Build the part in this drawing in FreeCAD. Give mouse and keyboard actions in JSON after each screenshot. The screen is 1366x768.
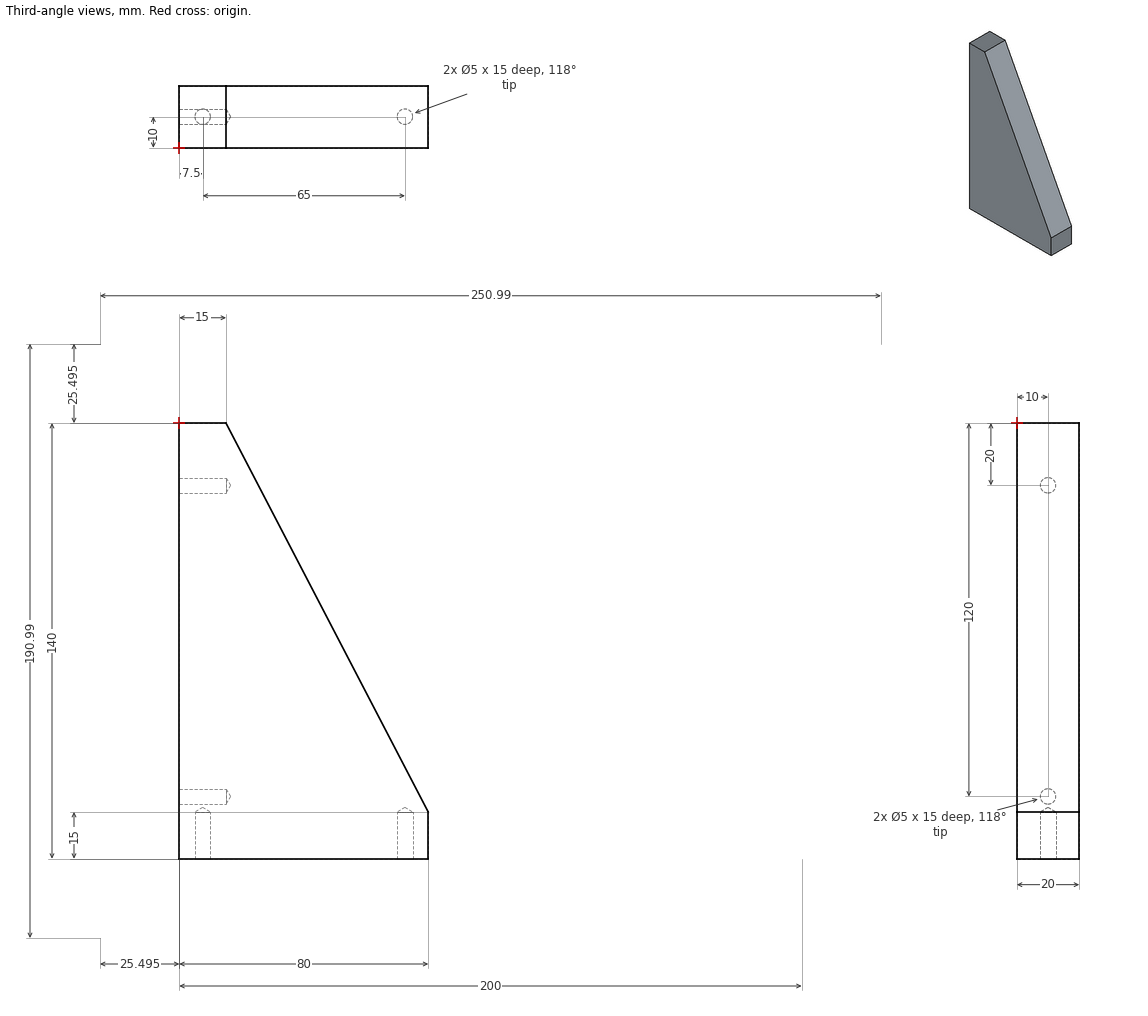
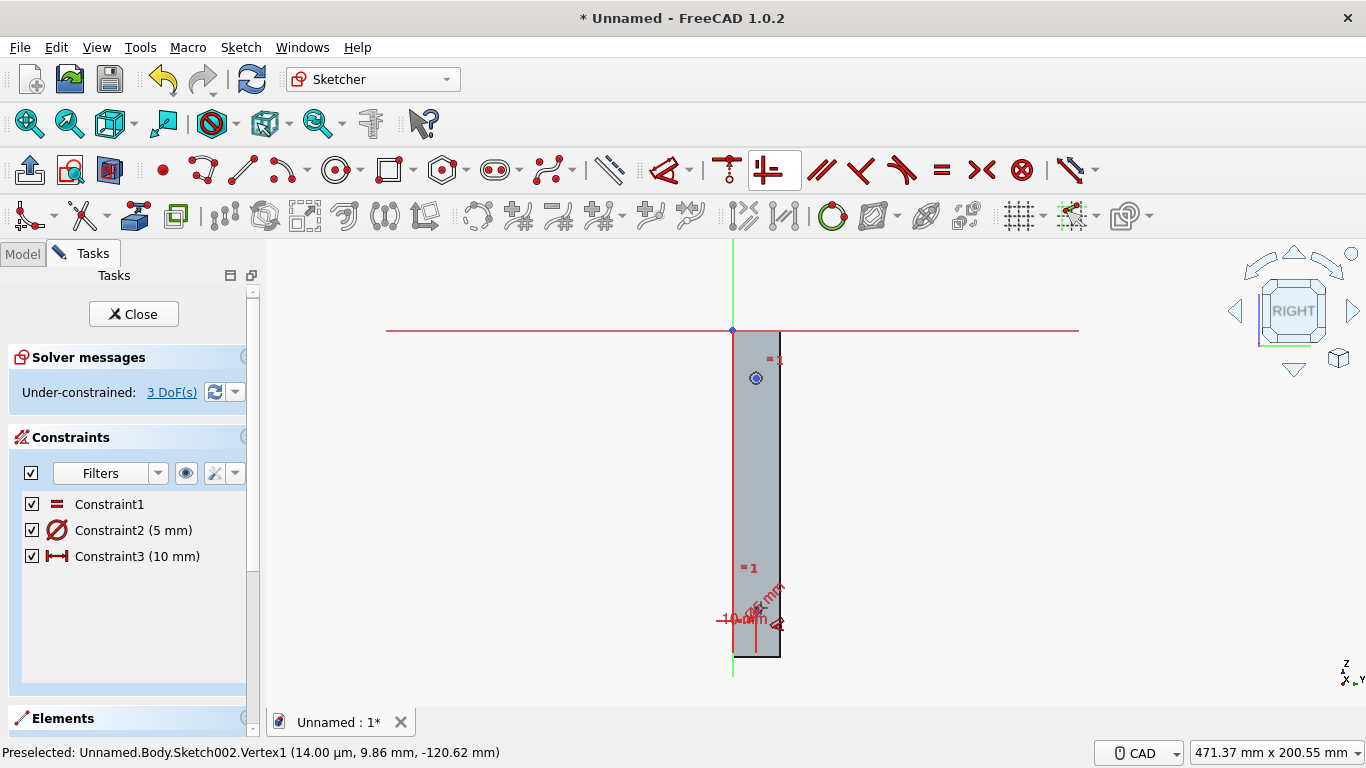
{"action": "scroll", "coordinate": [756, 378], "scroll_direction": "up", "scroll_amount": 3}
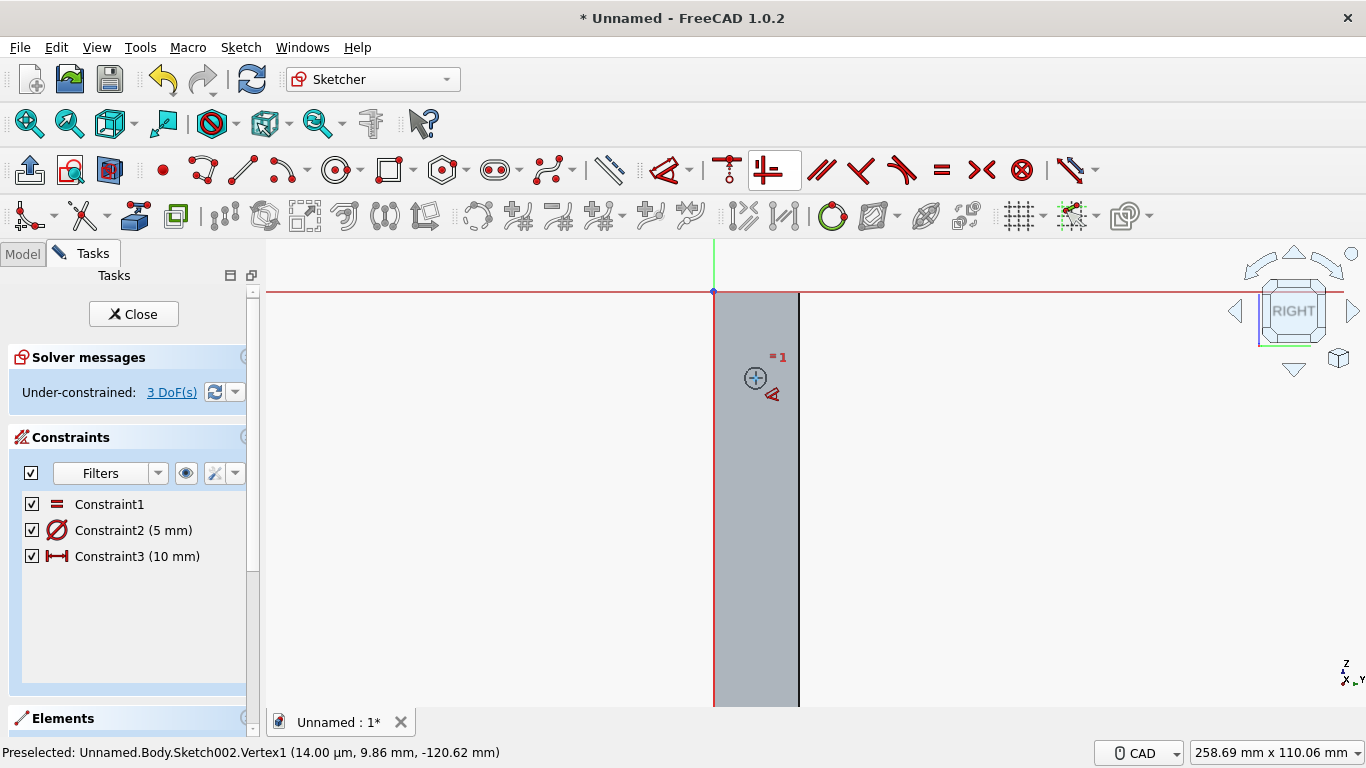
{"action": "left_click", "coordinate": [756, 378]}
{"action": "left_click", "coordinate": [735, 412]}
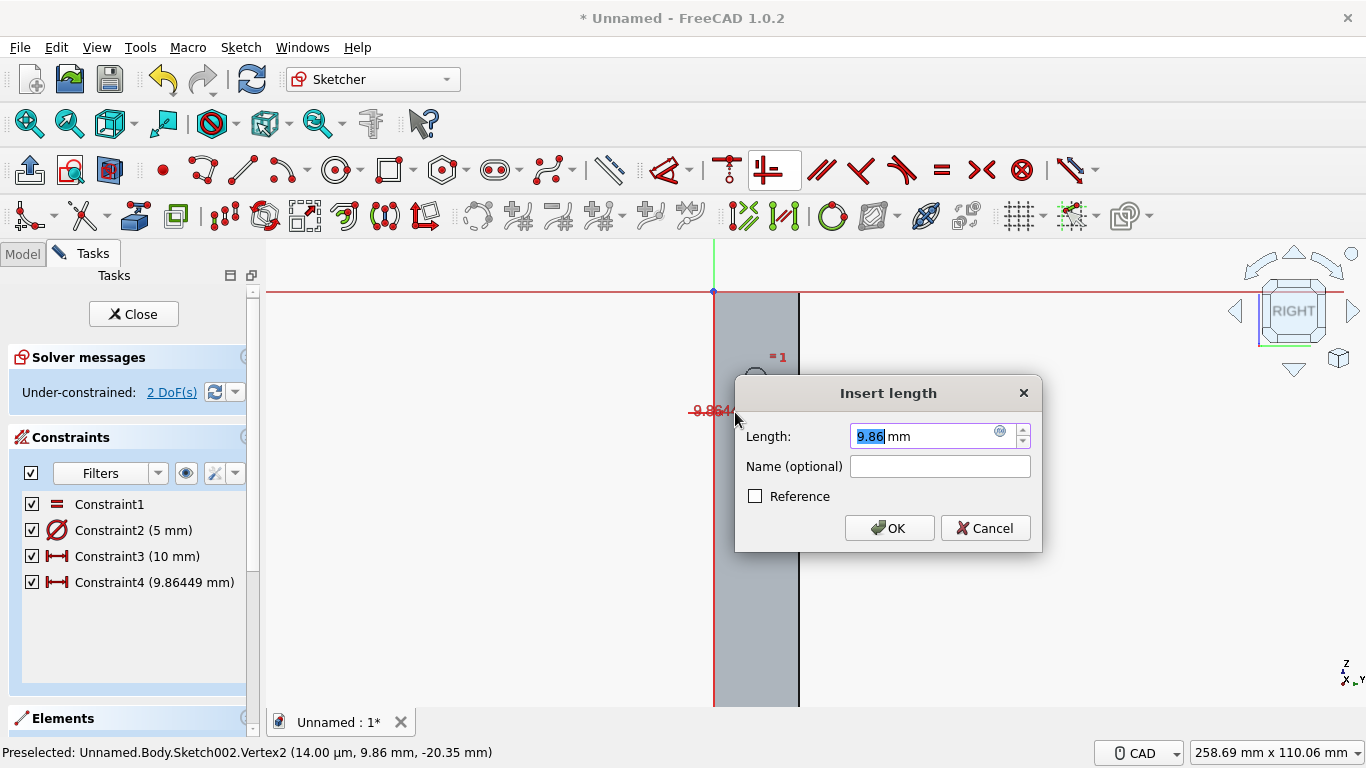
{"action": "type", "text": "10"}
{"action": "key", "text": "Return"}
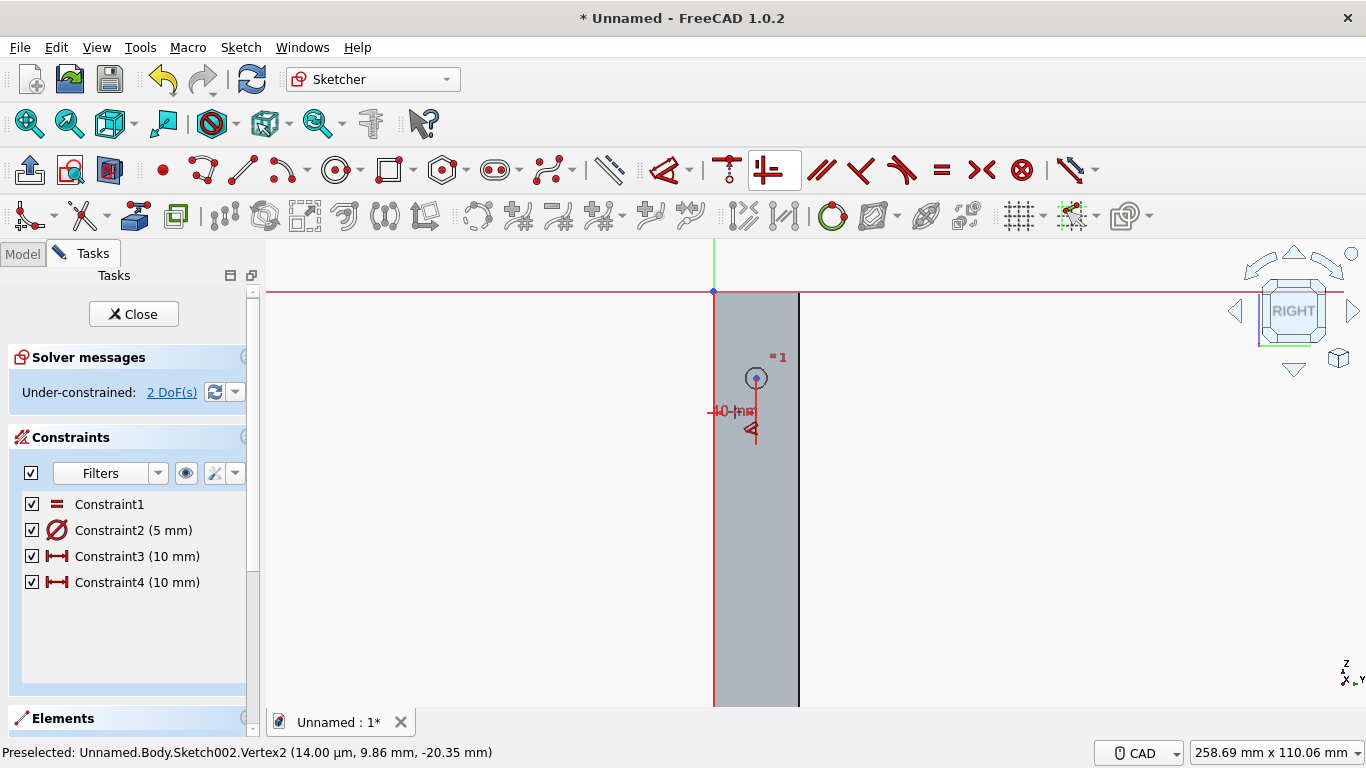
{"action": "left_click", "coordinate": [756, 378]}
{"action": "left_click", "coordinate": [680, 335]}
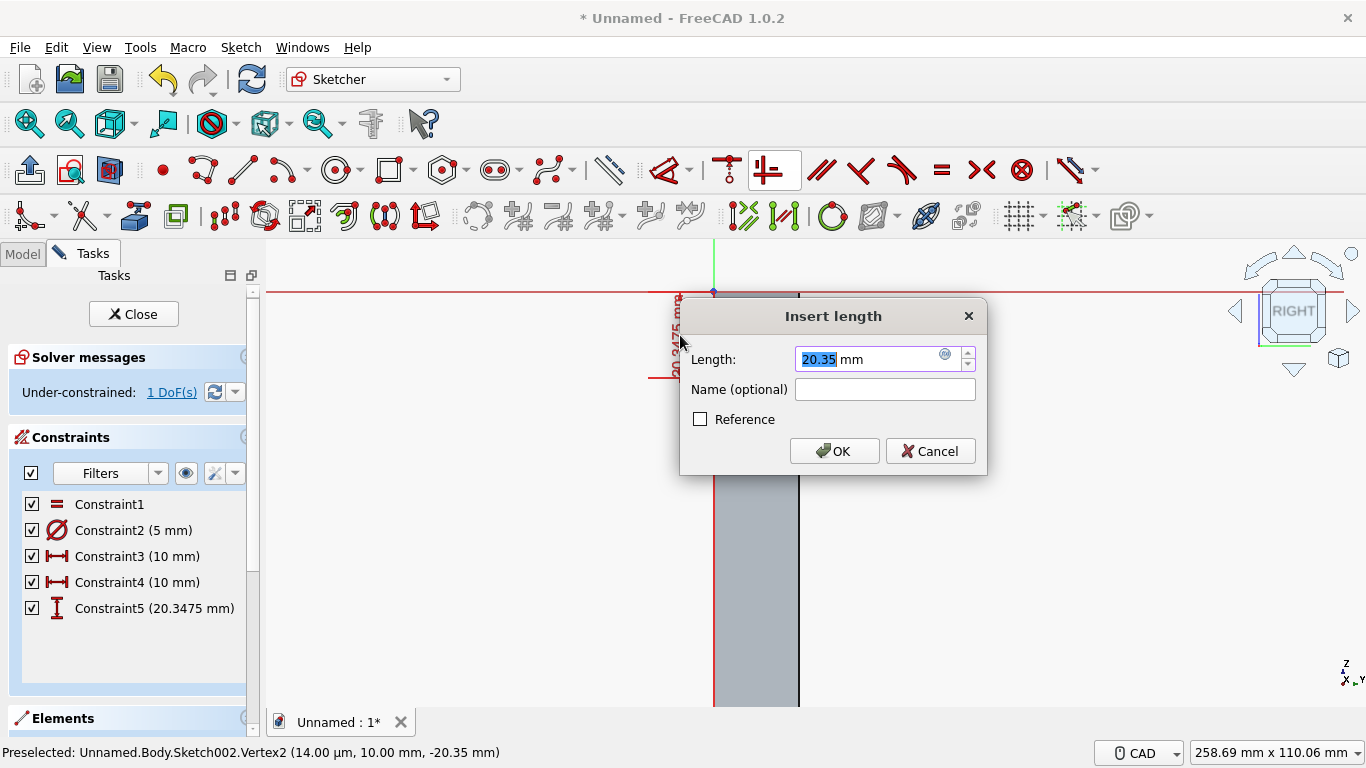
{"action": "type", "text": "20"}
{"action": "key", "text": "Return"}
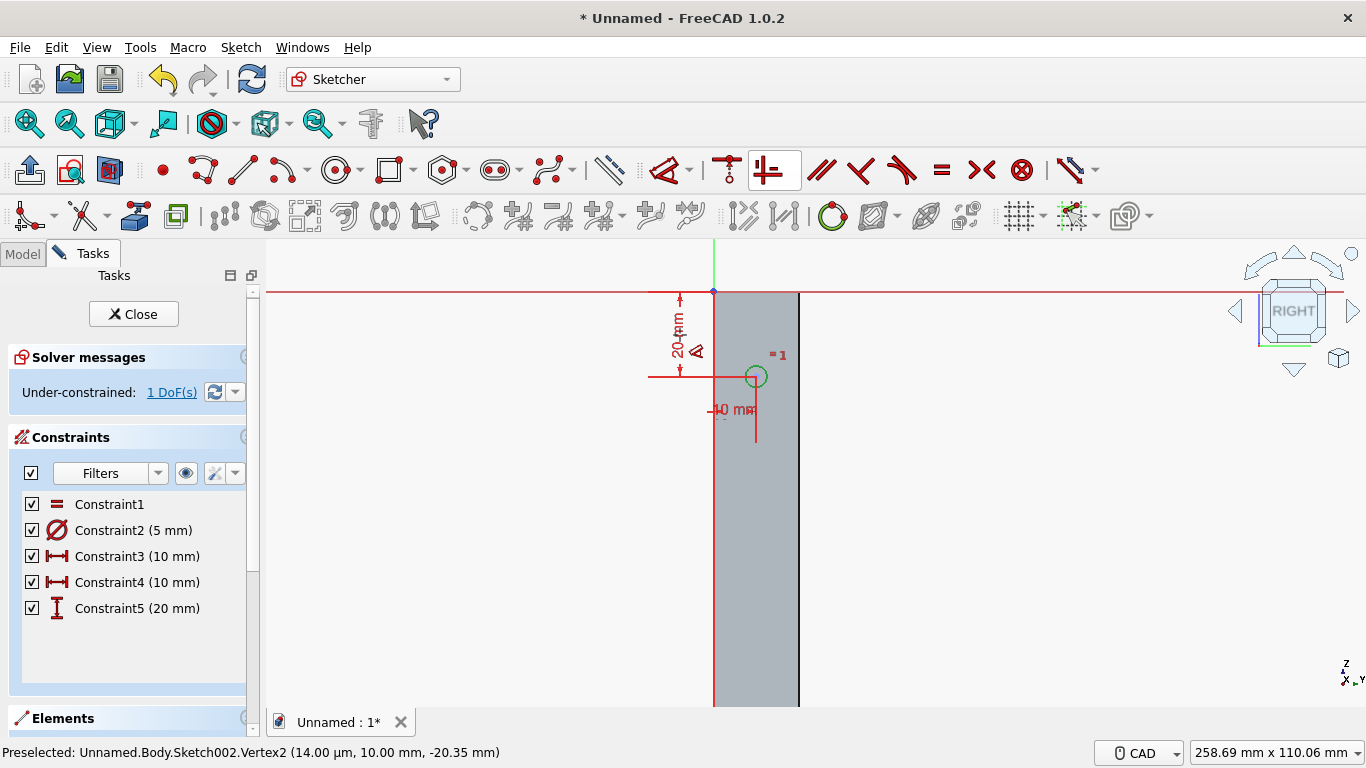
{"action": "scroll", "coordinate": [756, 377], "scroll_direction": "down", "scroll_amount": 3}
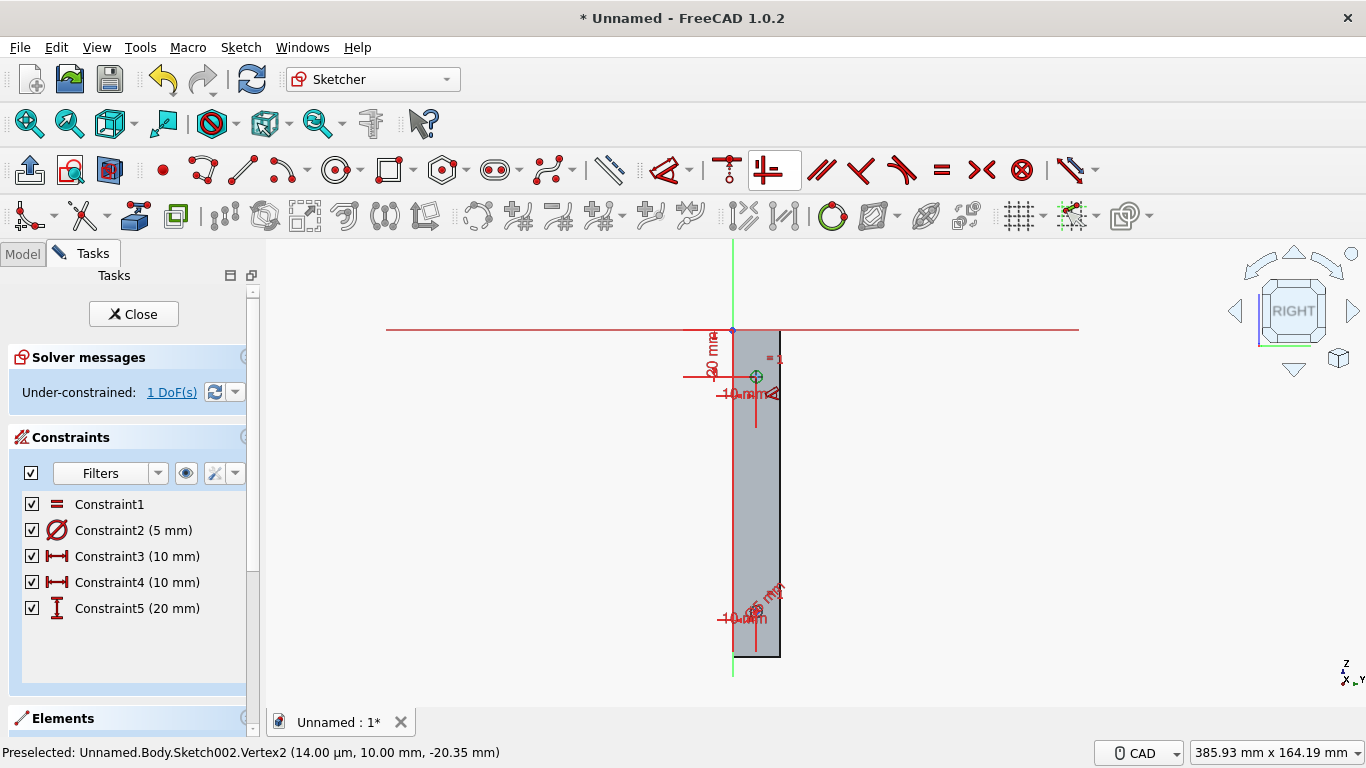
{"action": "left_click", "coordinate": [756, 612]}
{"action": "left_click", "coordinate": [699, 471]}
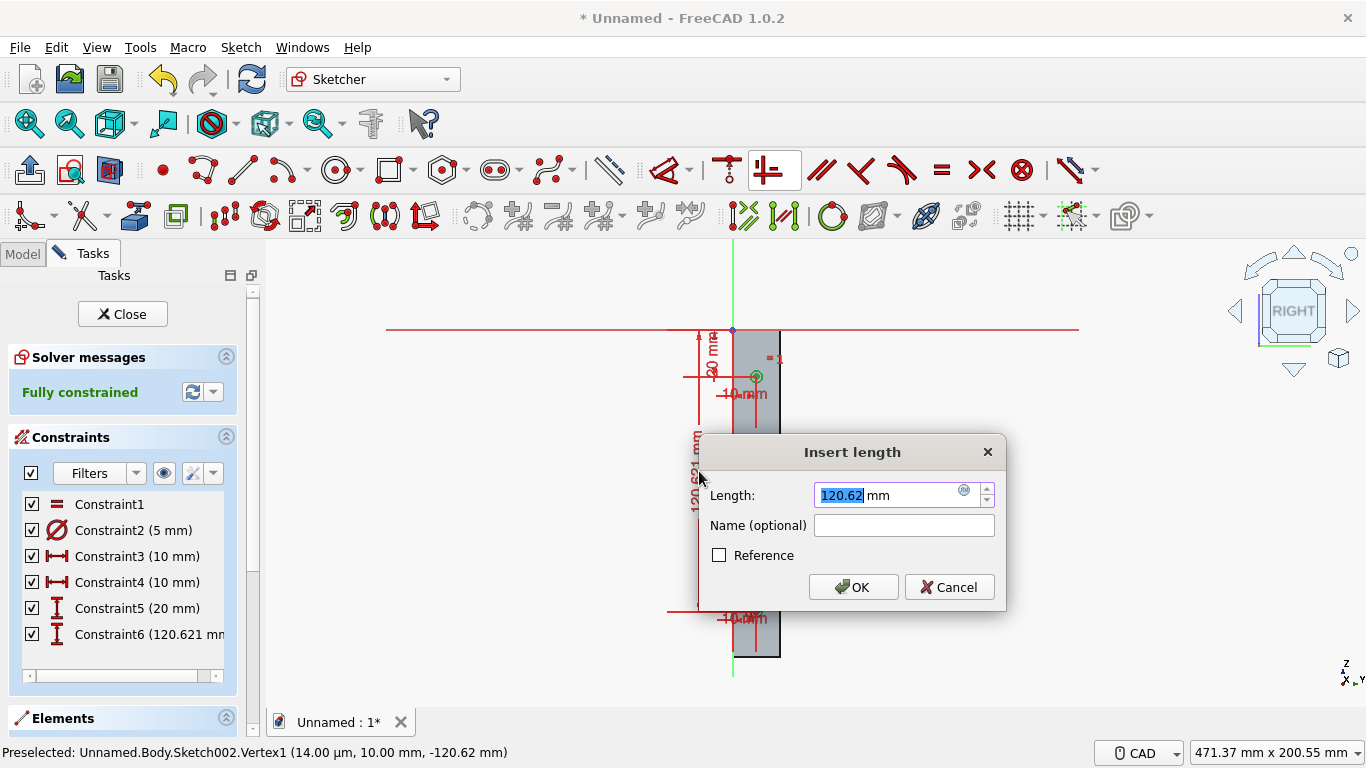
{"action": "type", "text": "120"}
{"action": "key", "text": "Return"}
{"action": "key", "text": "Escape"}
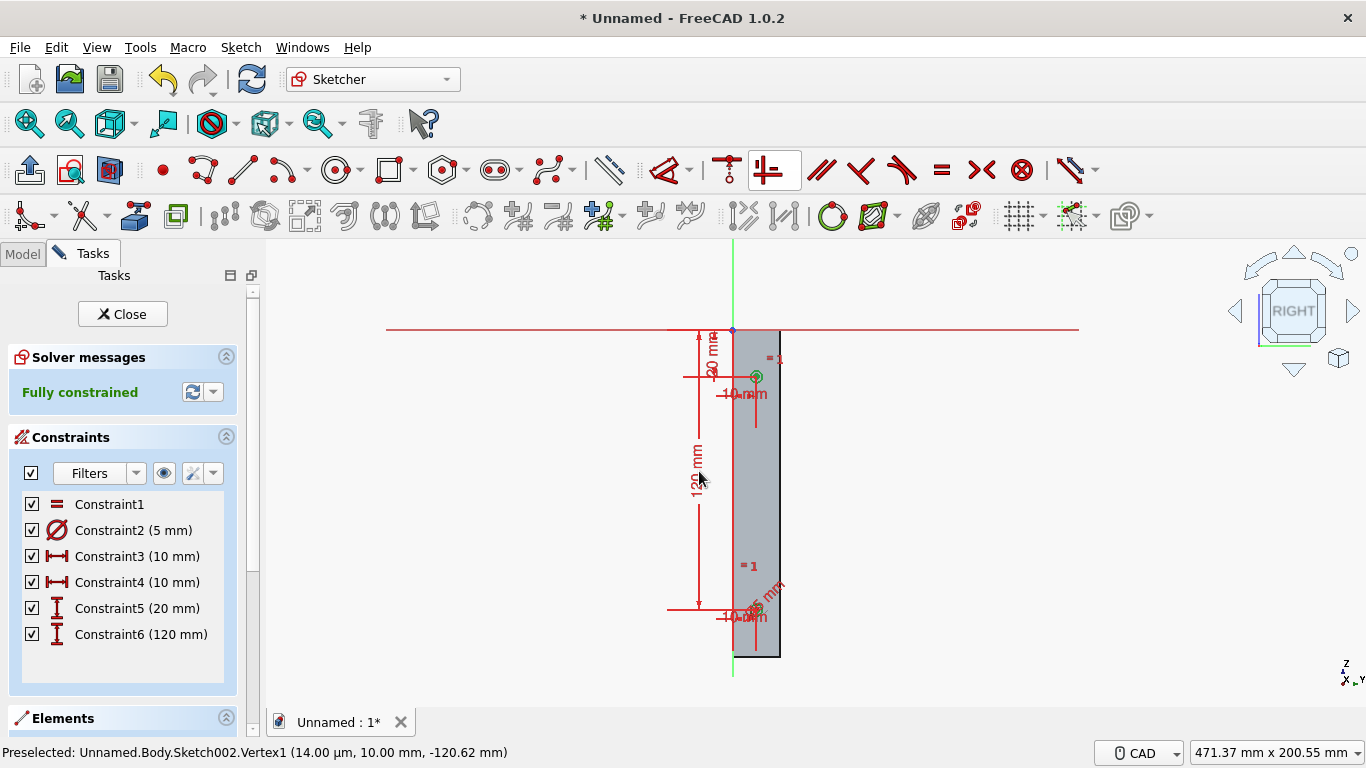
{"action": "left_click", "coordinate": [123, 314]}